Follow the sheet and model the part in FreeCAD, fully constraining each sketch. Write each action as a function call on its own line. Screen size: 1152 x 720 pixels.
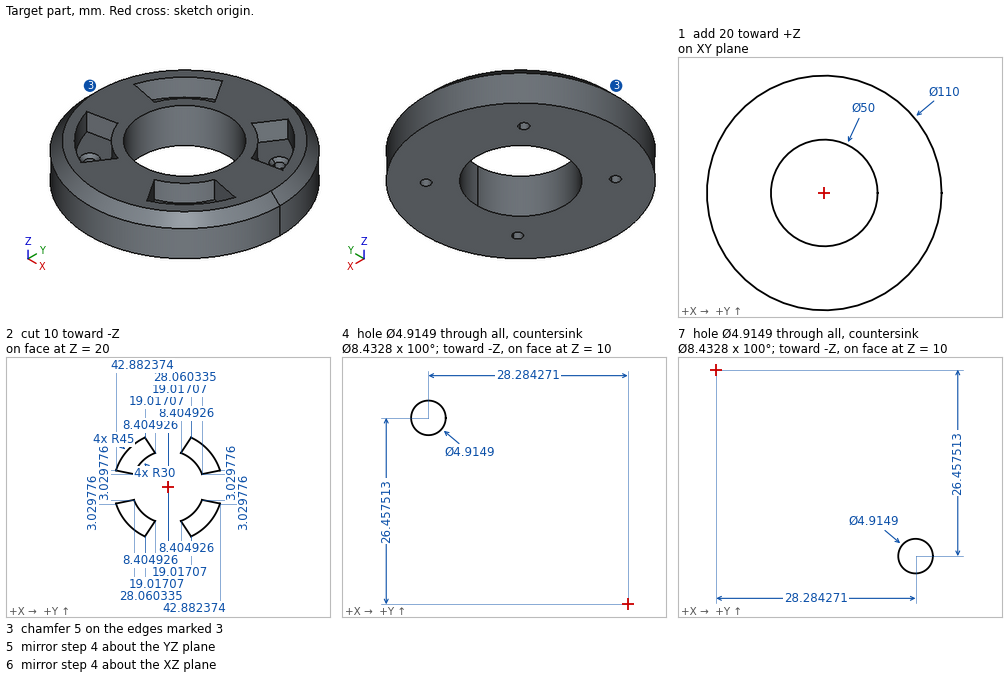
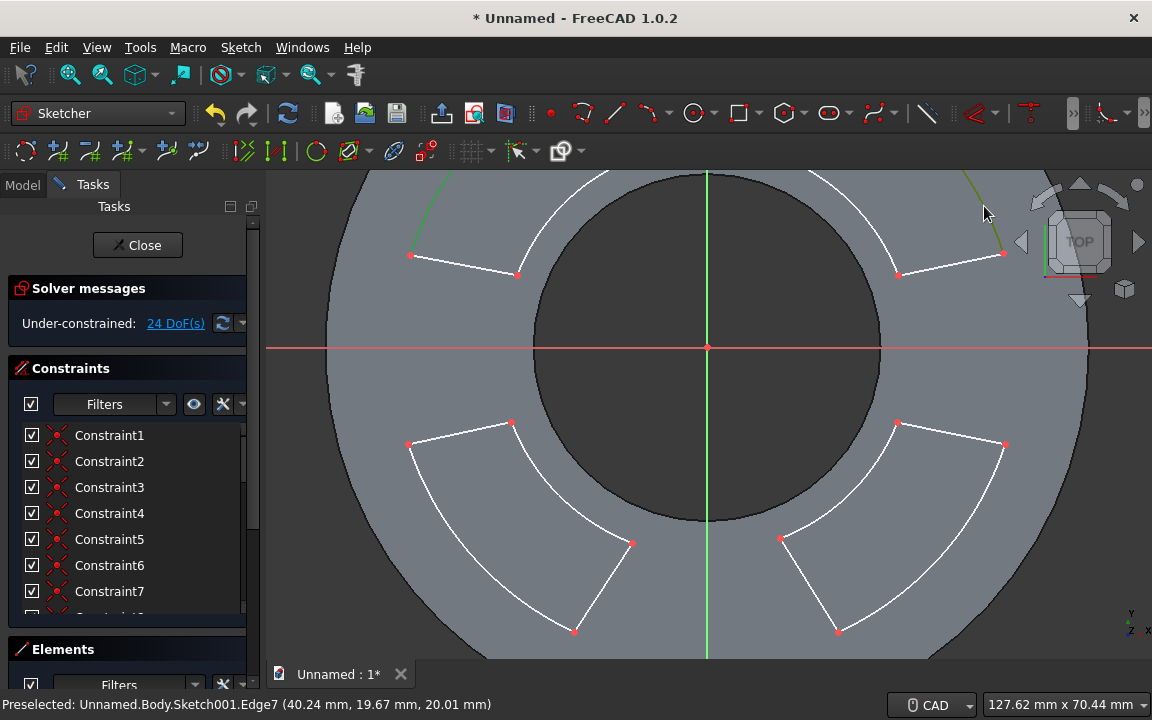
click(904, 591)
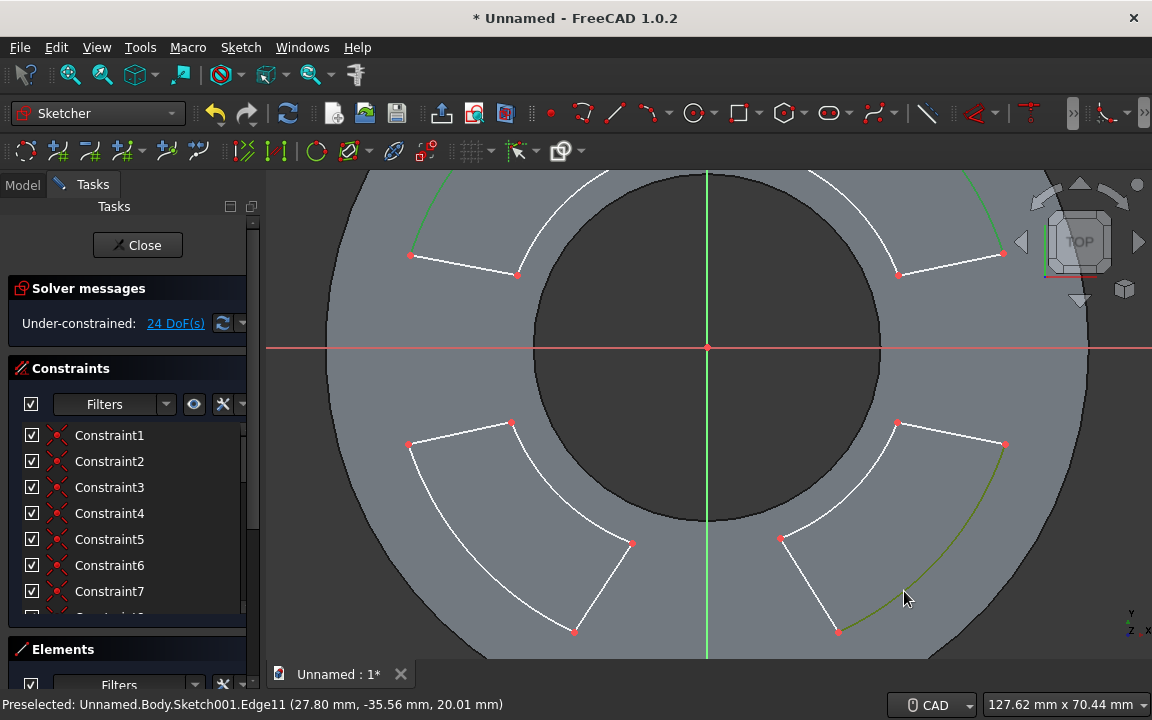
click(441, 514)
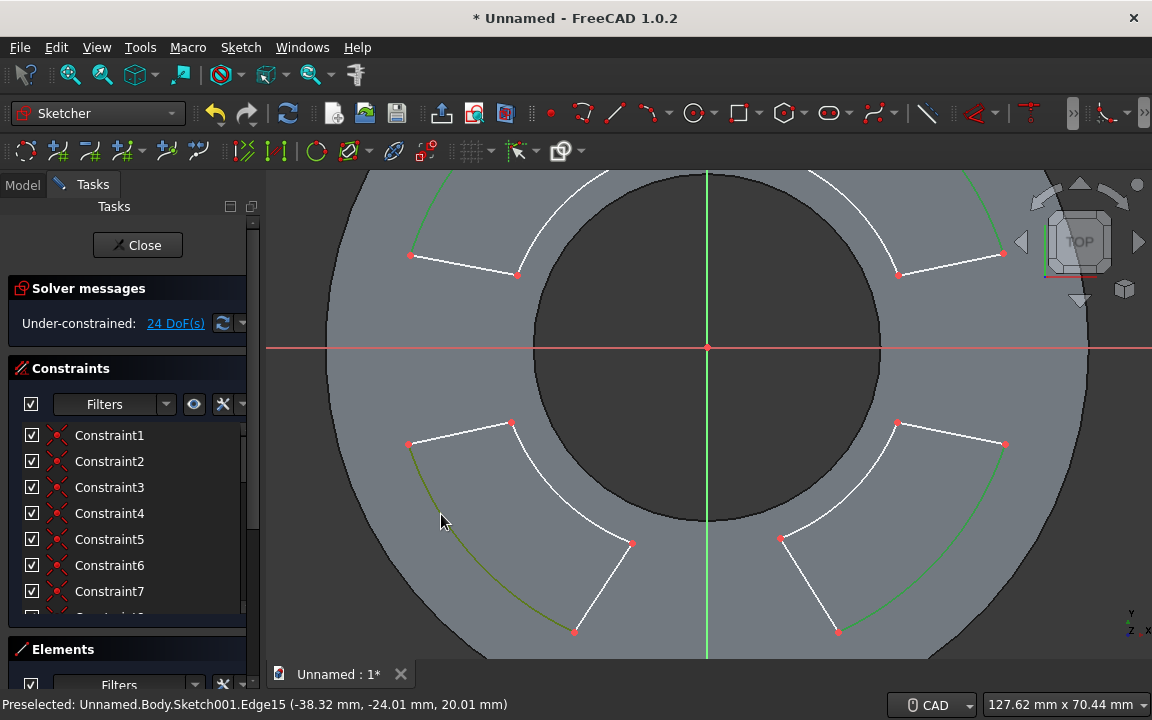
key(e)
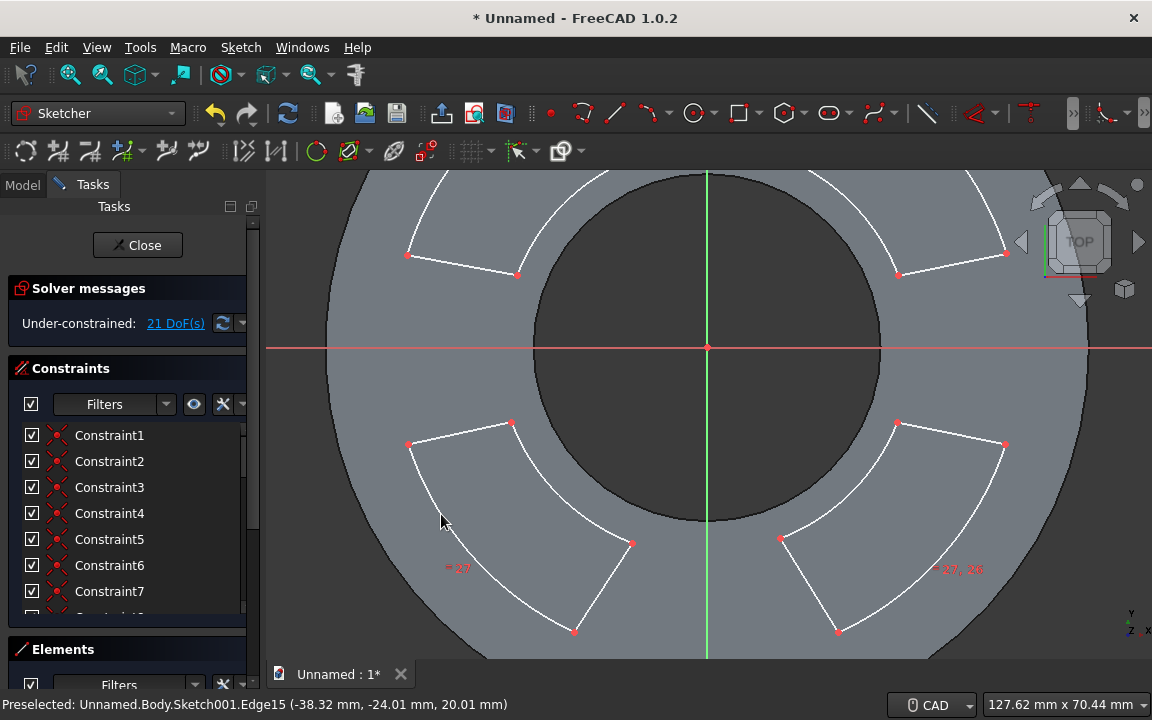
click(541, 230)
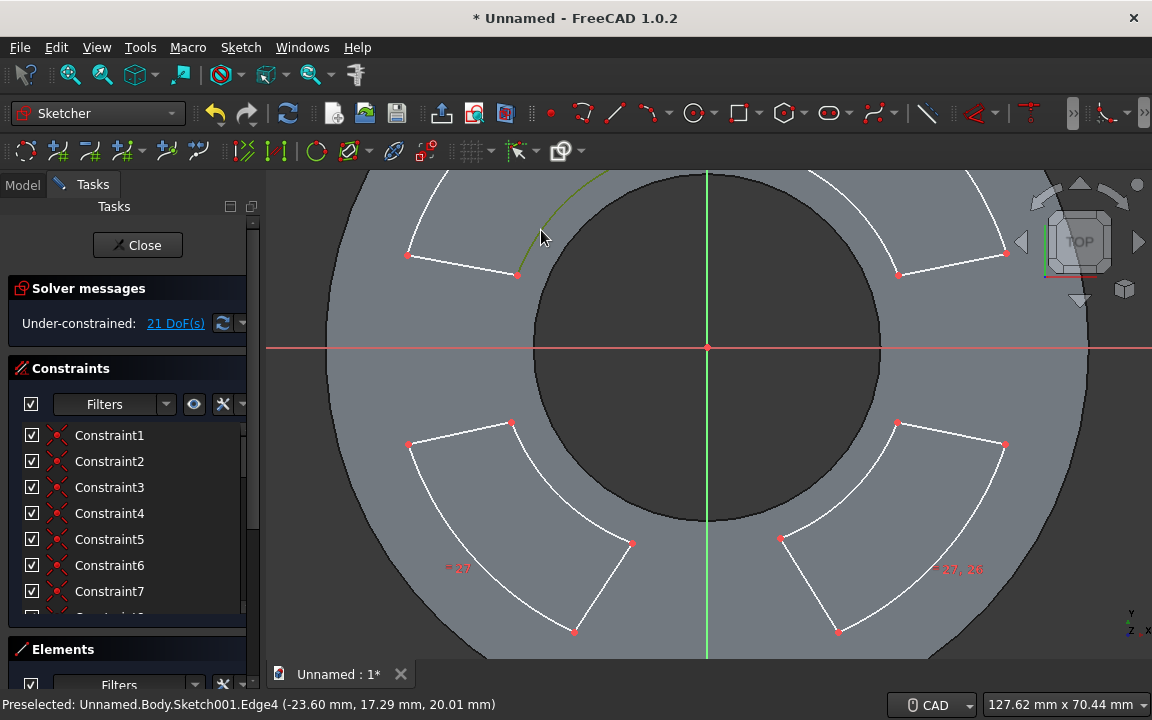
click(874, 230)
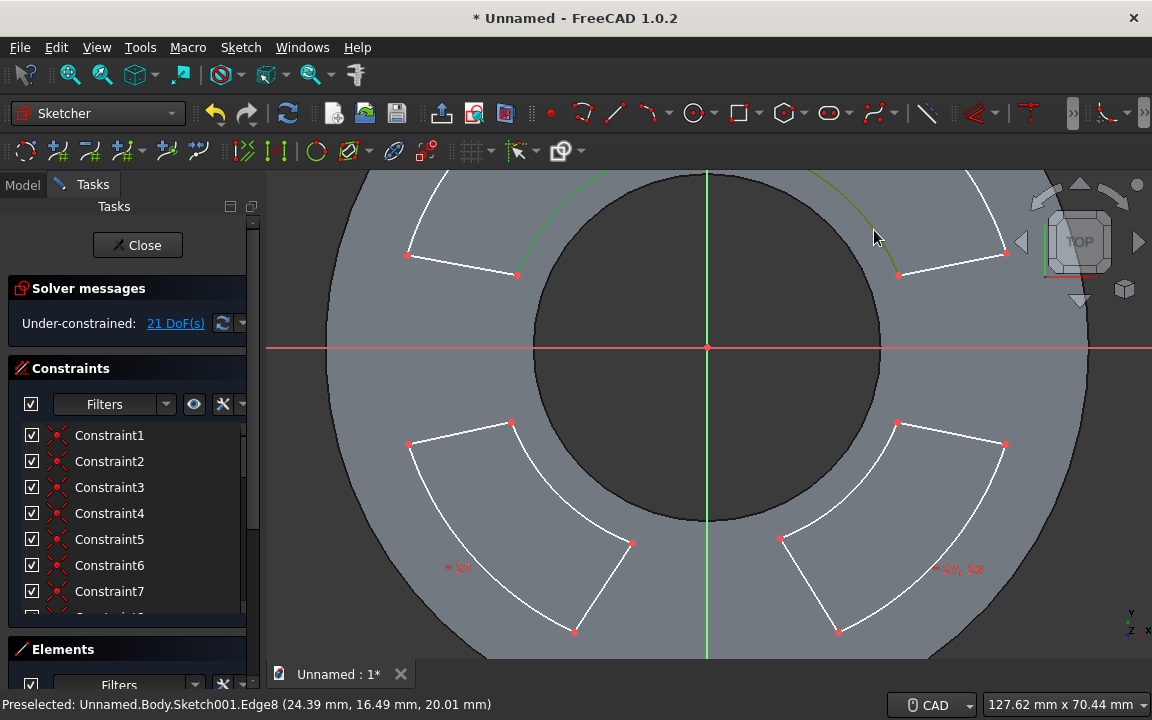
click(825, 515)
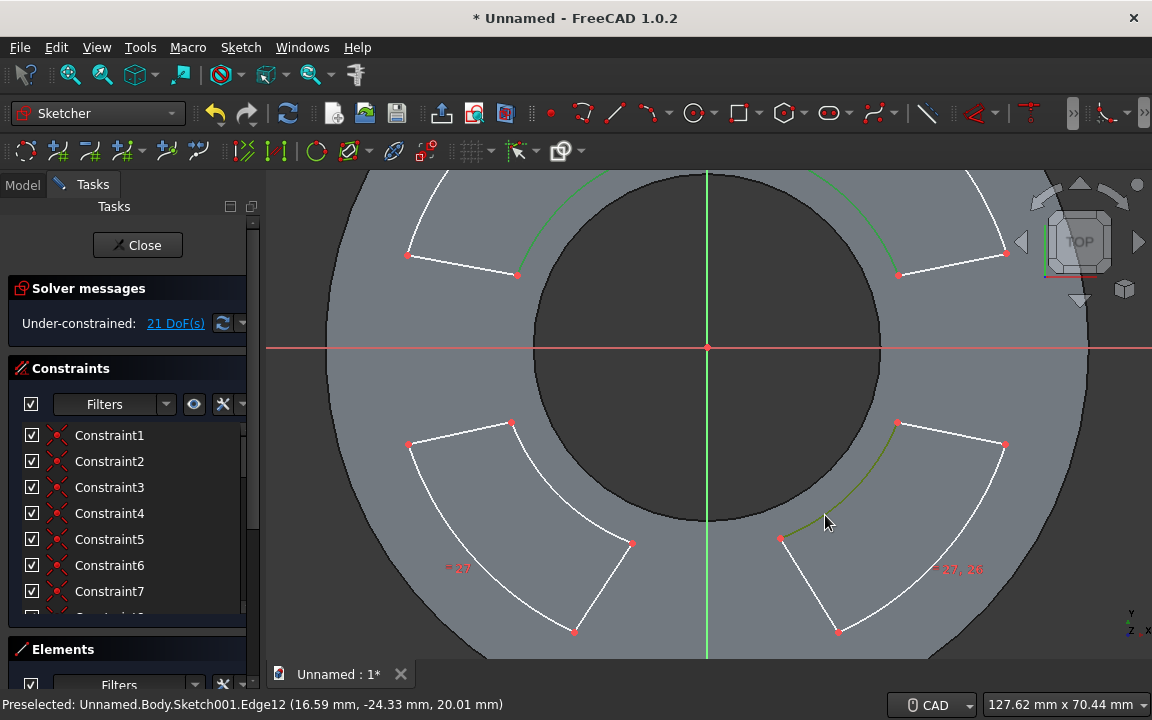
click(536, 469)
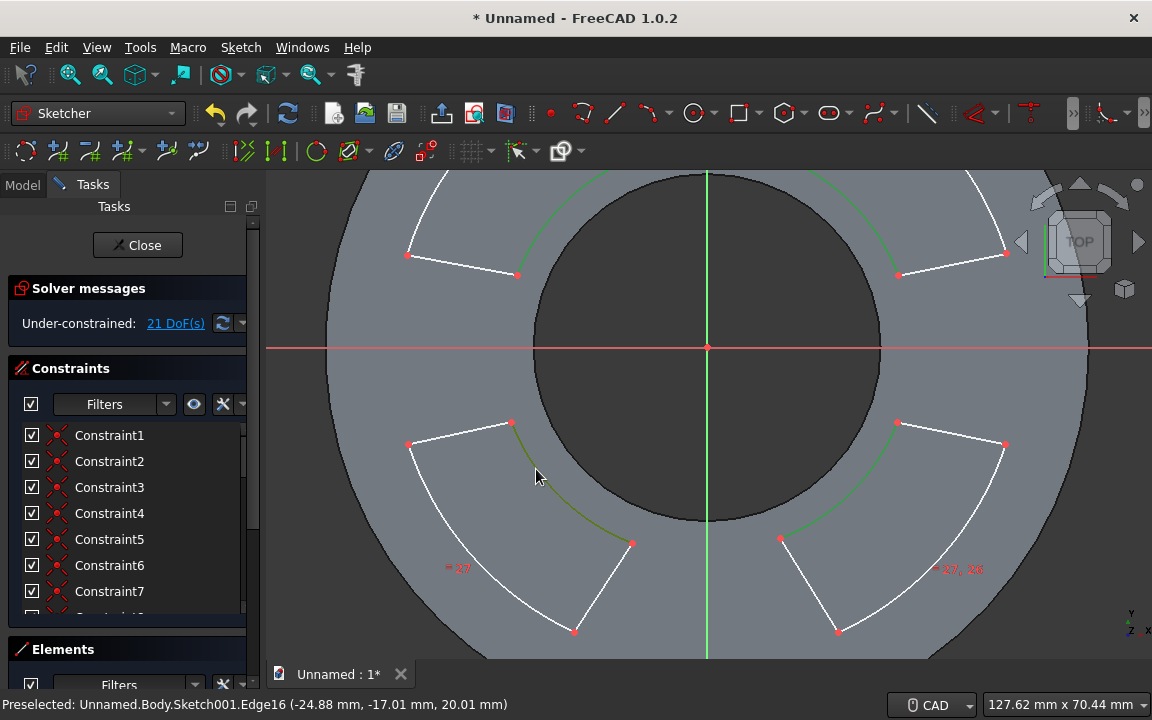
key(e)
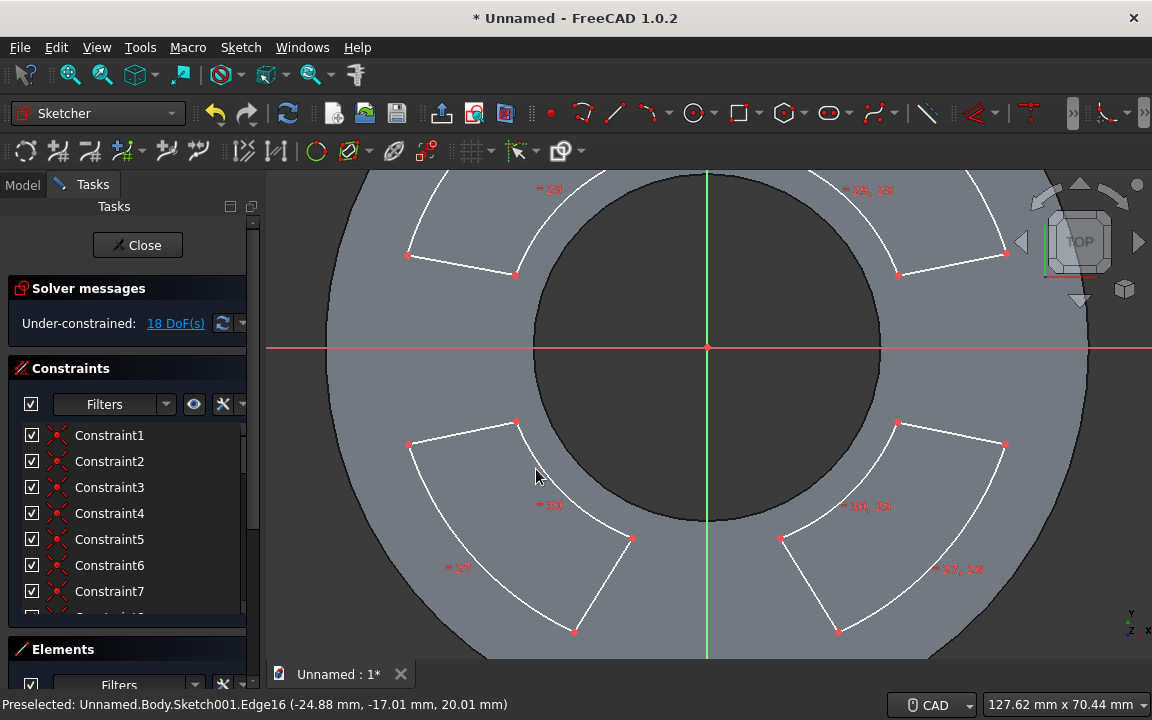
click(974, 114)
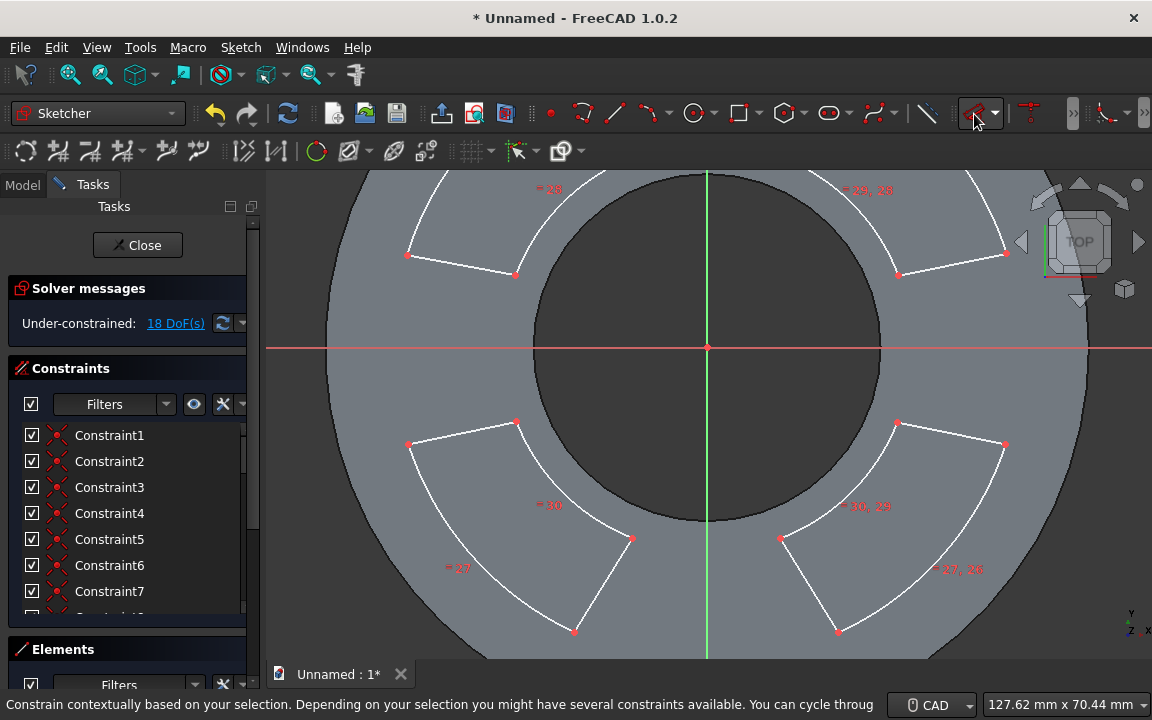
click(427, 206)
click(409, 523)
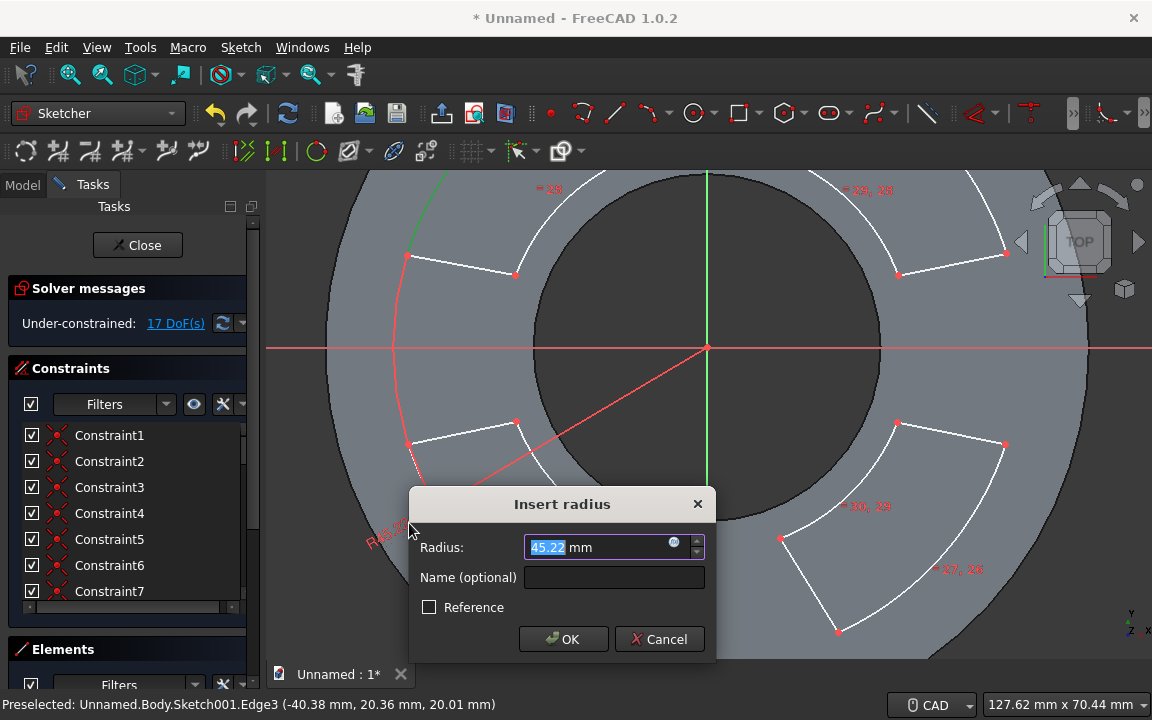
text(45)
key(Return)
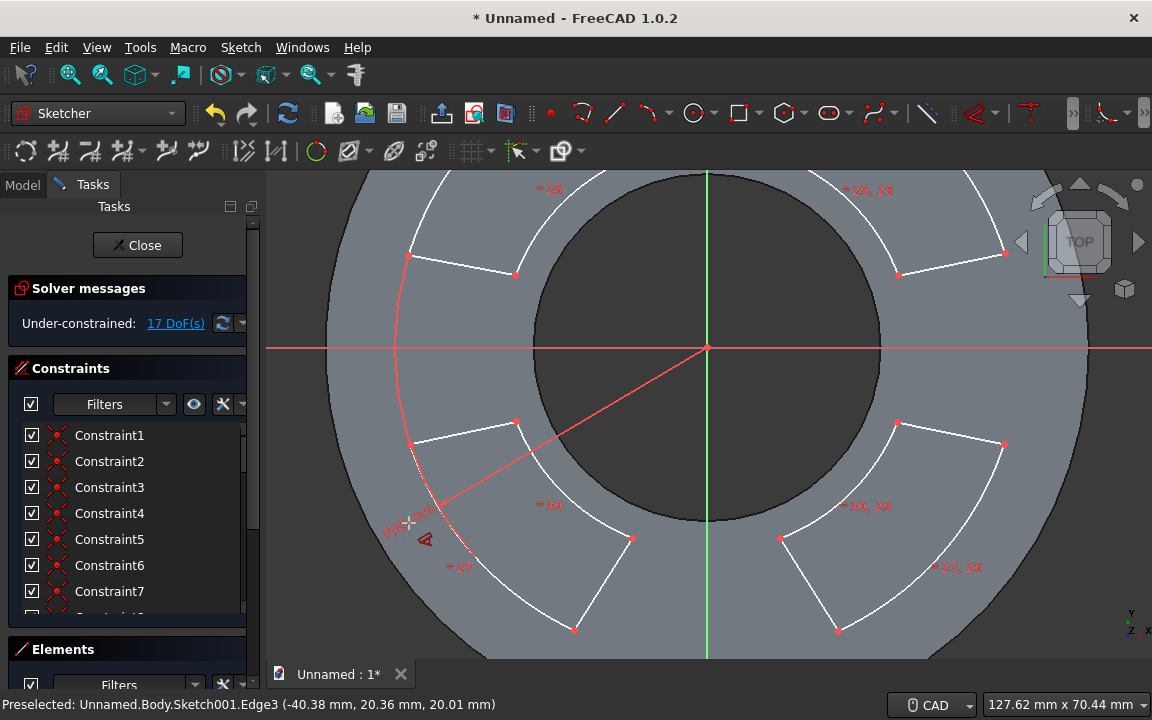
click(540, 230)
click(514, 212)